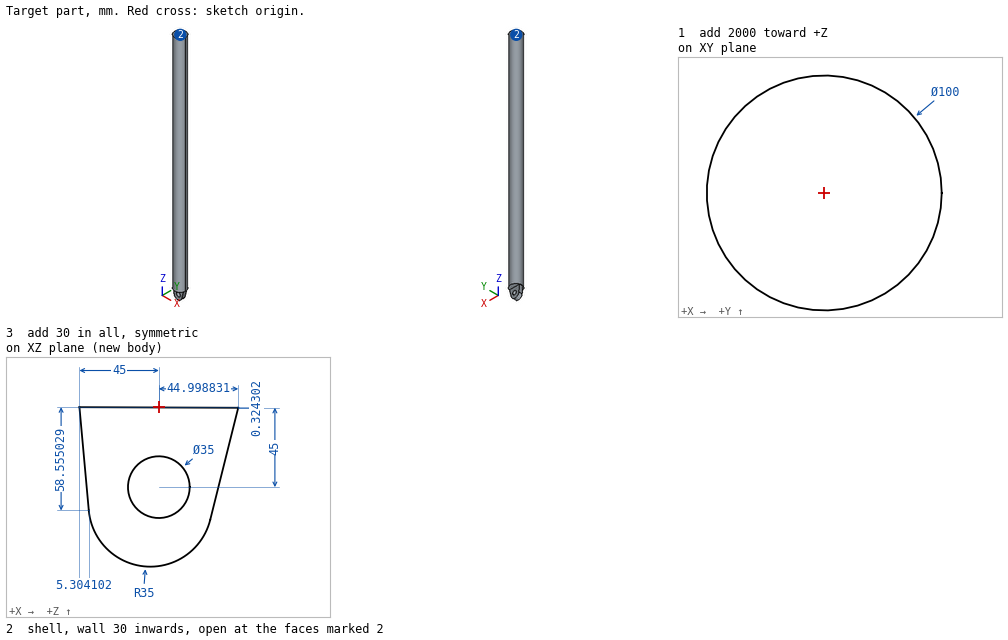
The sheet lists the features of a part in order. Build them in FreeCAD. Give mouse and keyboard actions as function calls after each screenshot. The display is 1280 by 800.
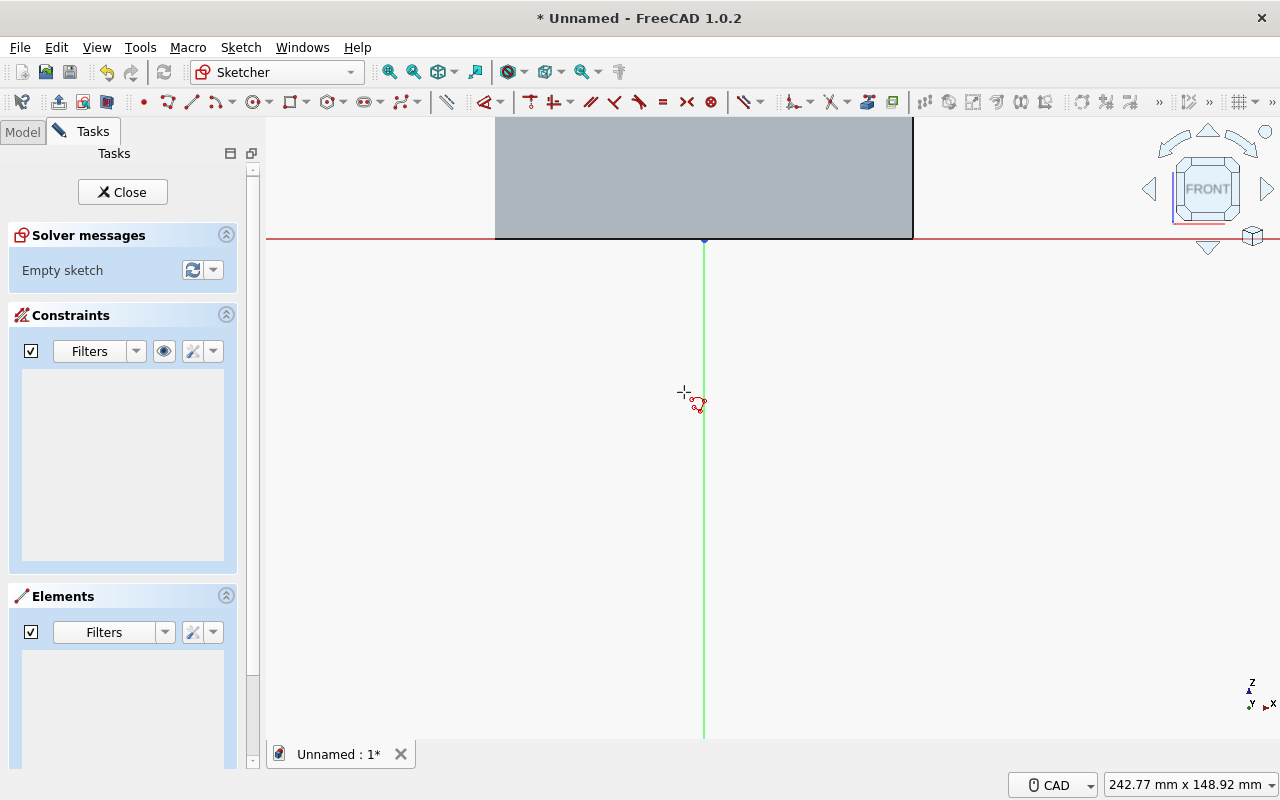
click(538, 484)
click(516, 239)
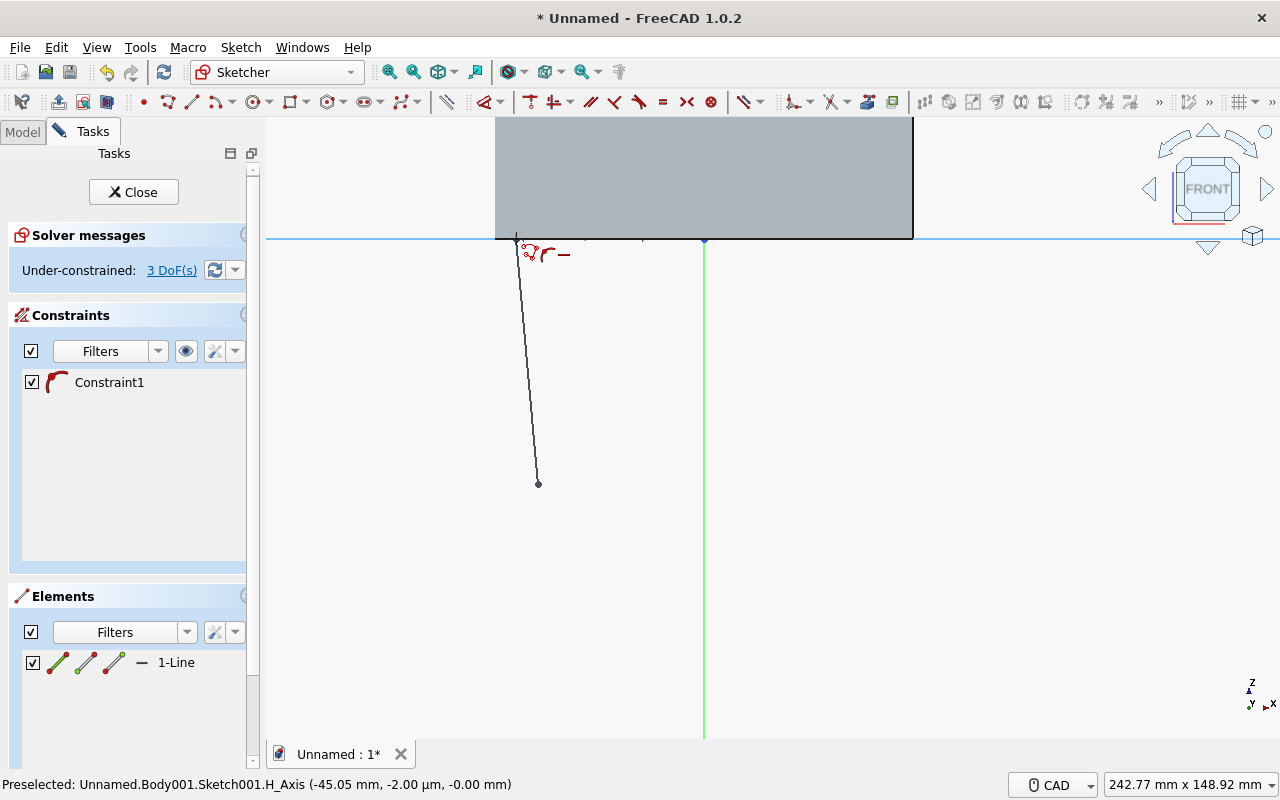
scroll(892, 241, up, 13)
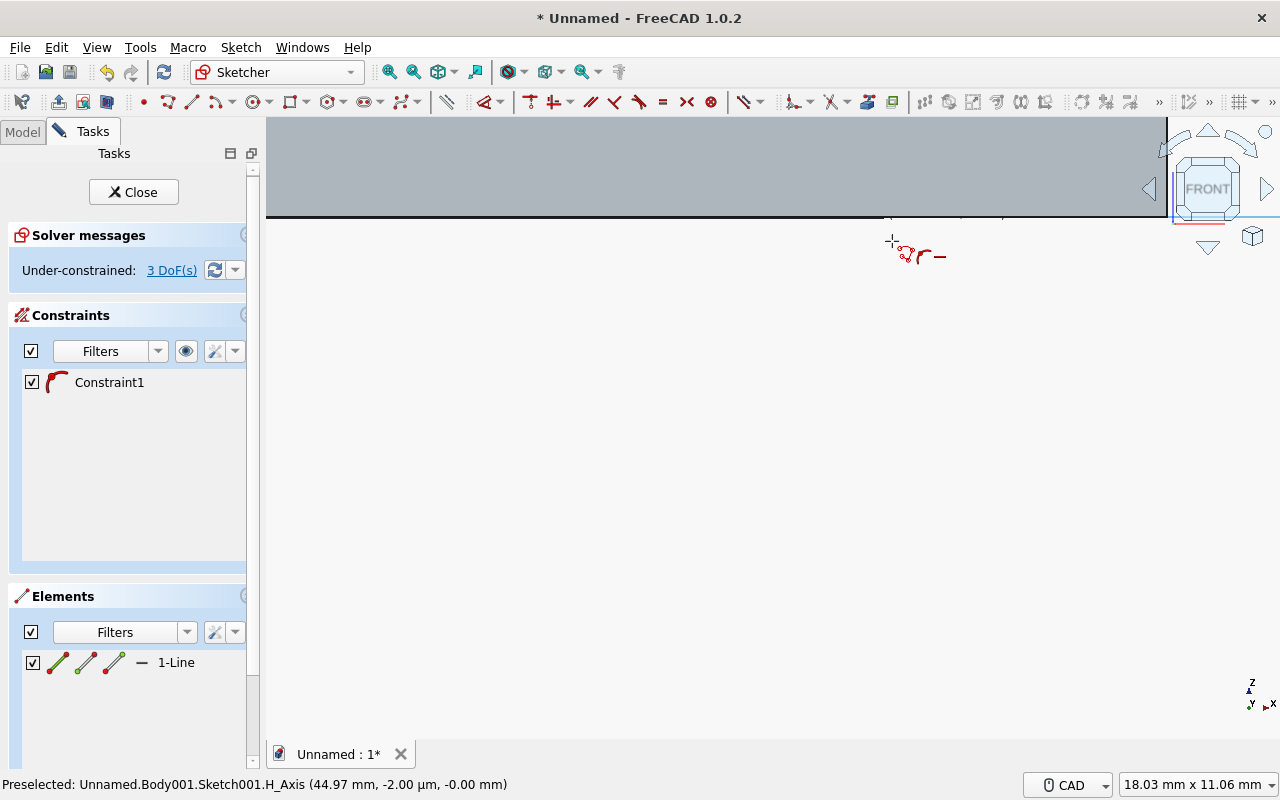
click(886, 447)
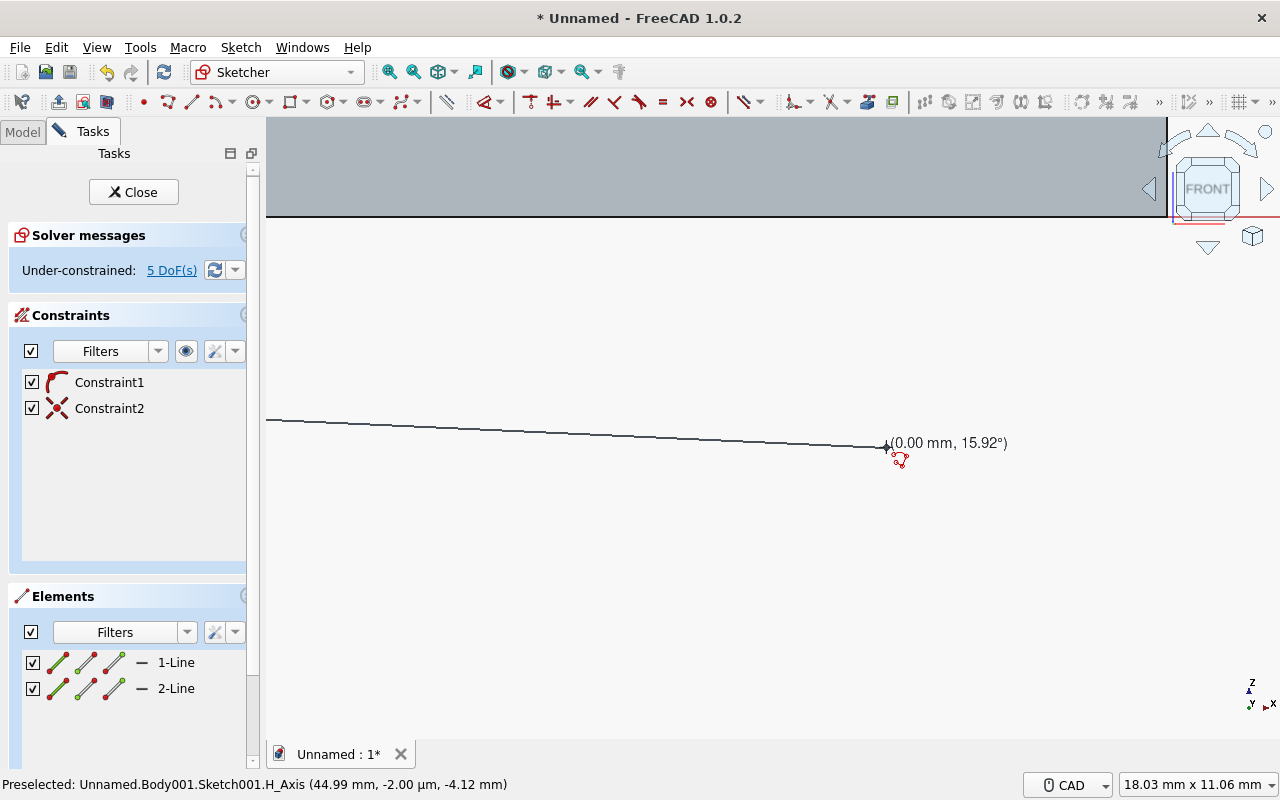
scroll(893, 241, down, 13)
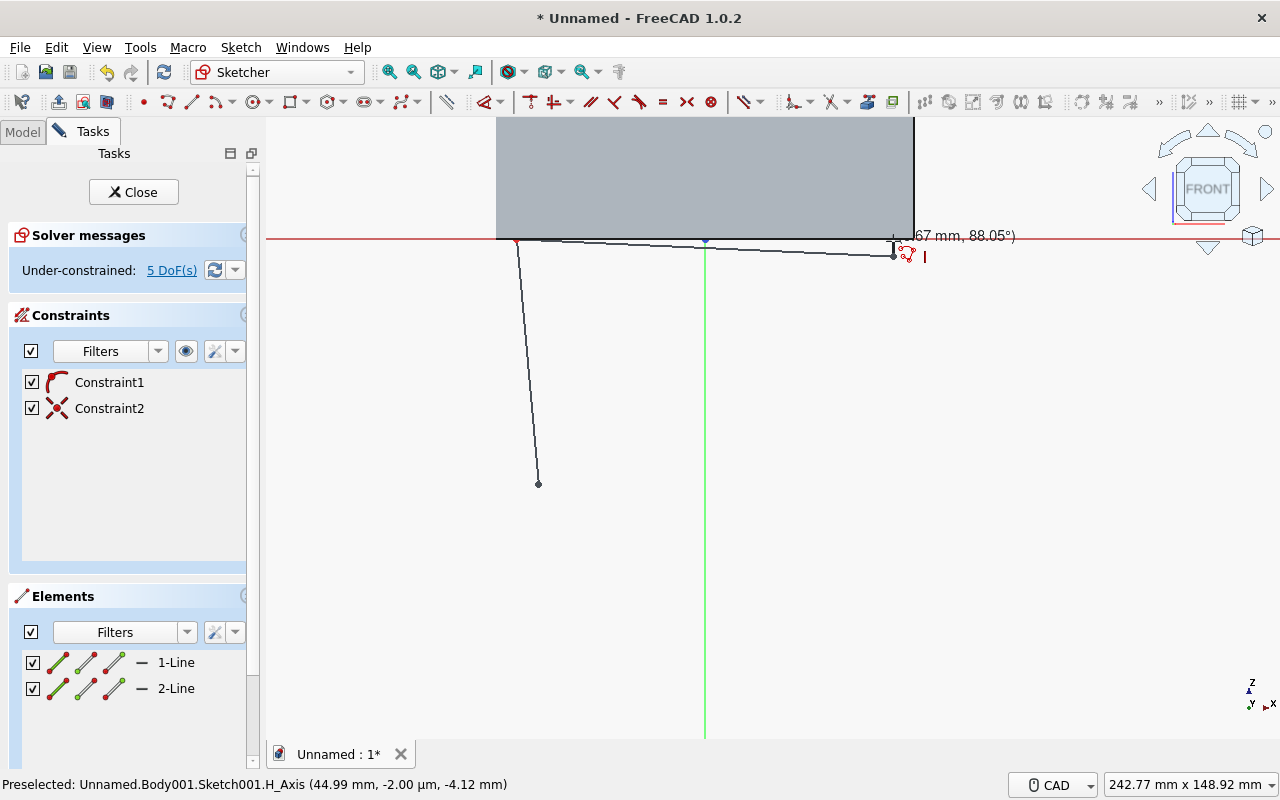
click(827, 506)
right_click(827, 506)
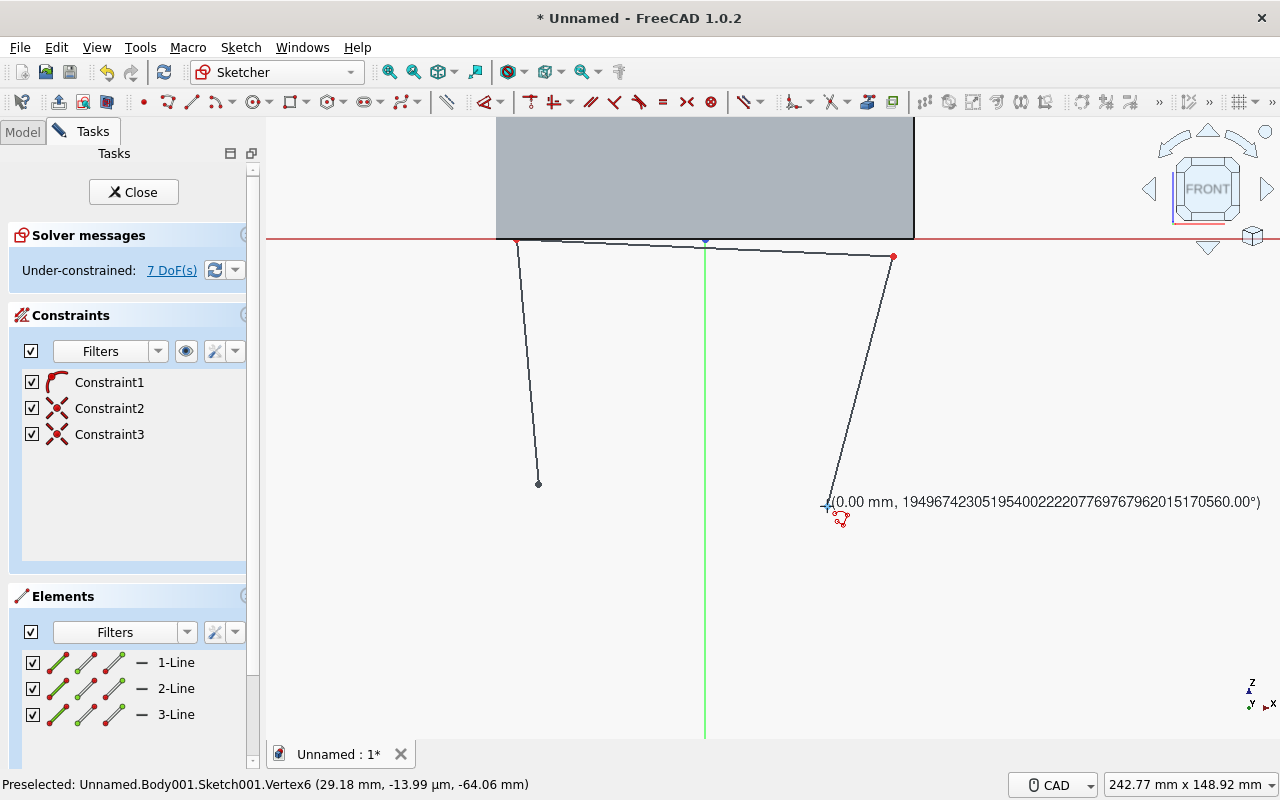
key(g)
key(3)
key(a)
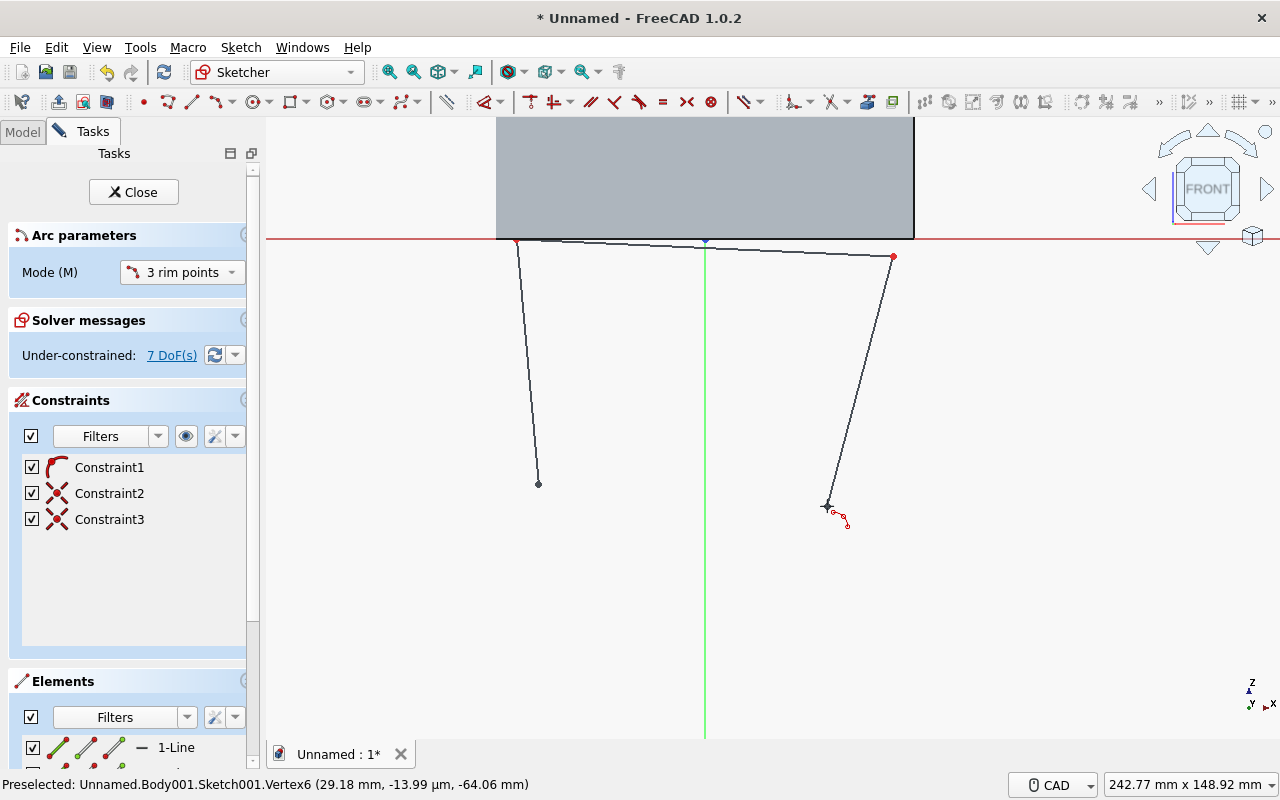
click(827, 507)
click(539, 485)
click(674, 617)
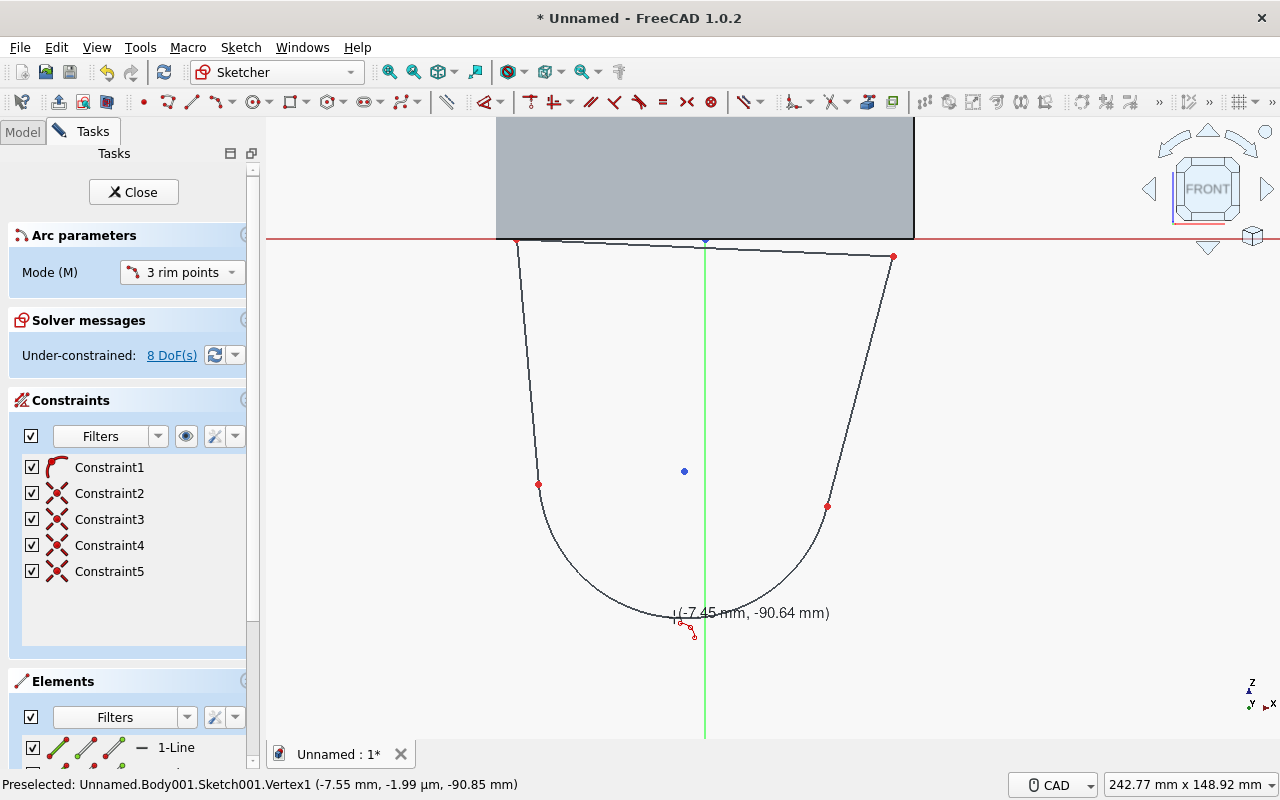
click(254, 102)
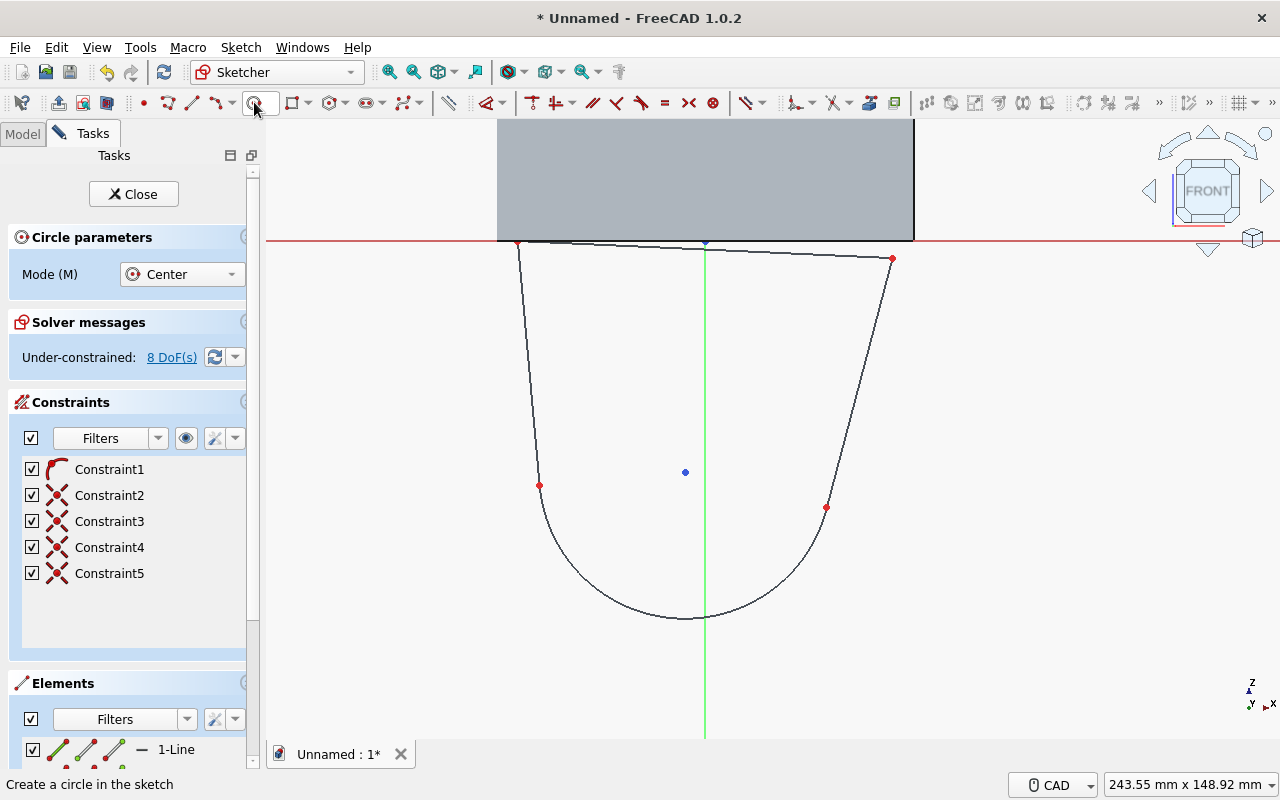
click(705, 430)
click(757, 378)
key(Escape)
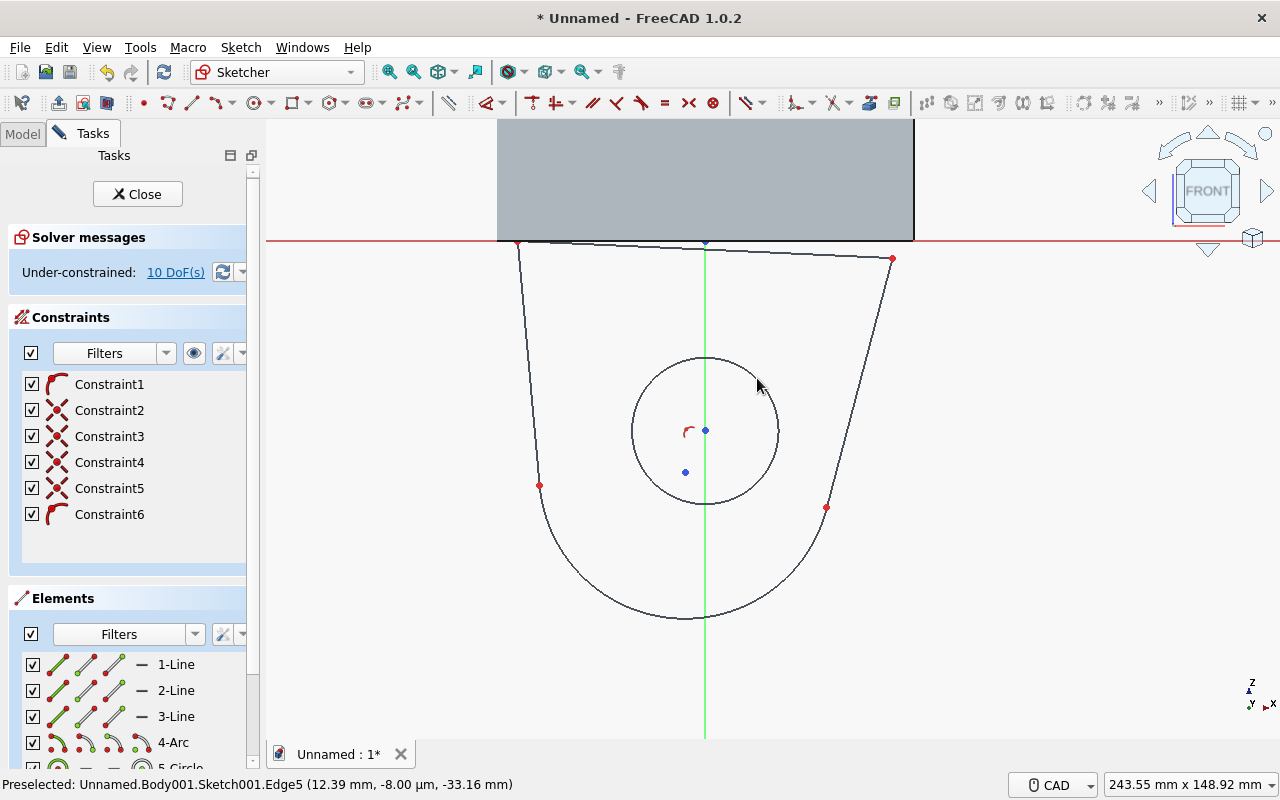
click(533, 412)